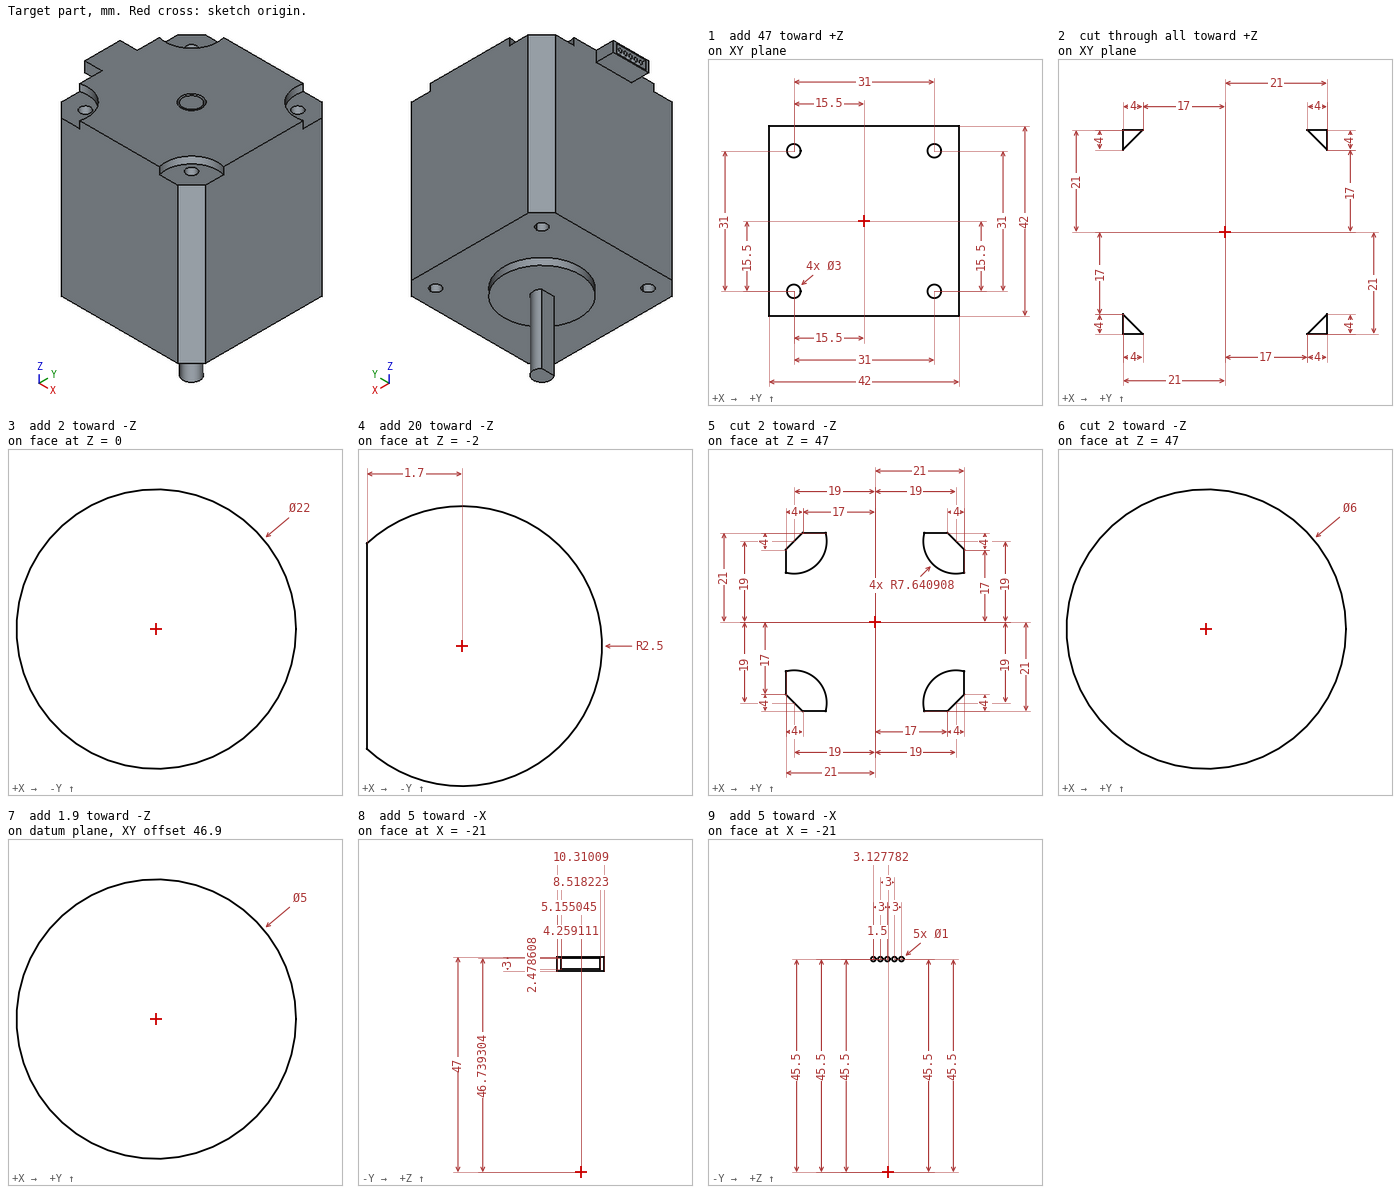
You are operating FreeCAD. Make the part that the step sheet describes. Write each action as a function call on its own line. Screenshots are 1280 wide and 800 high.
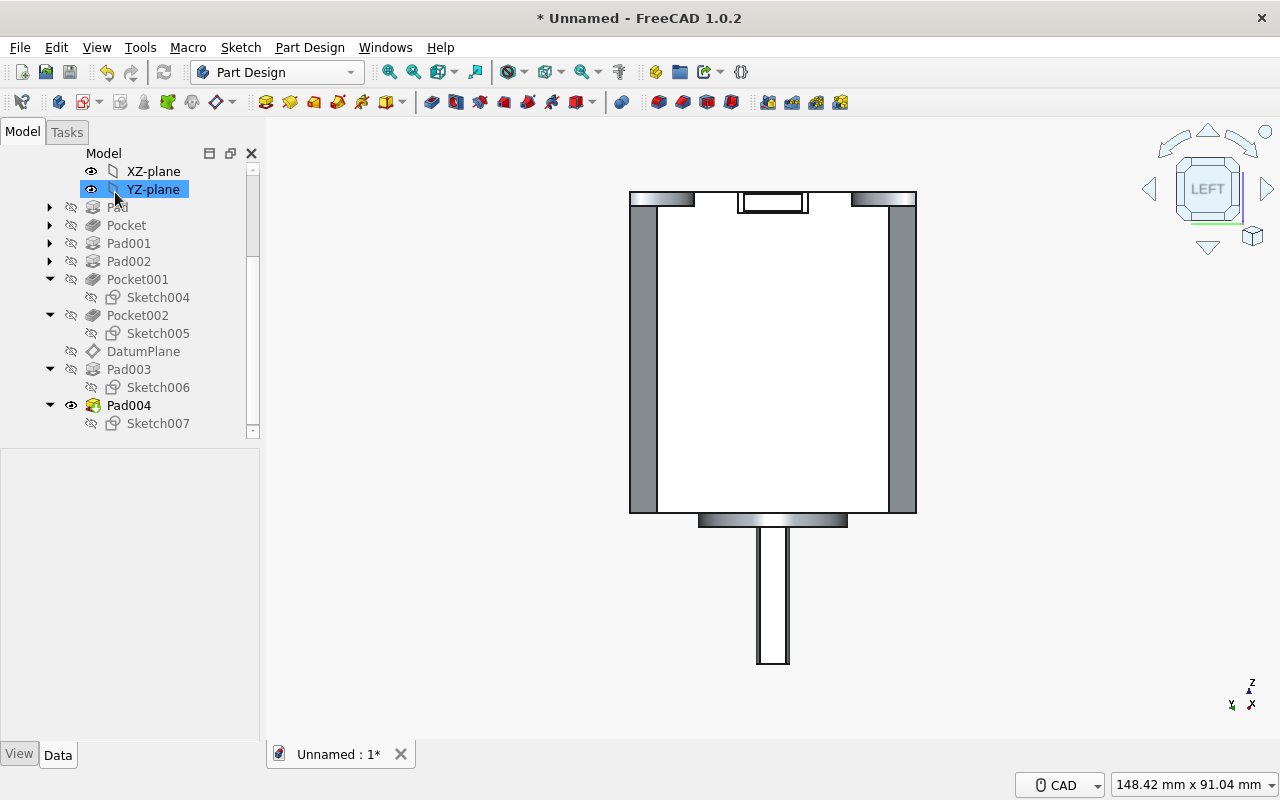
click(773, 352)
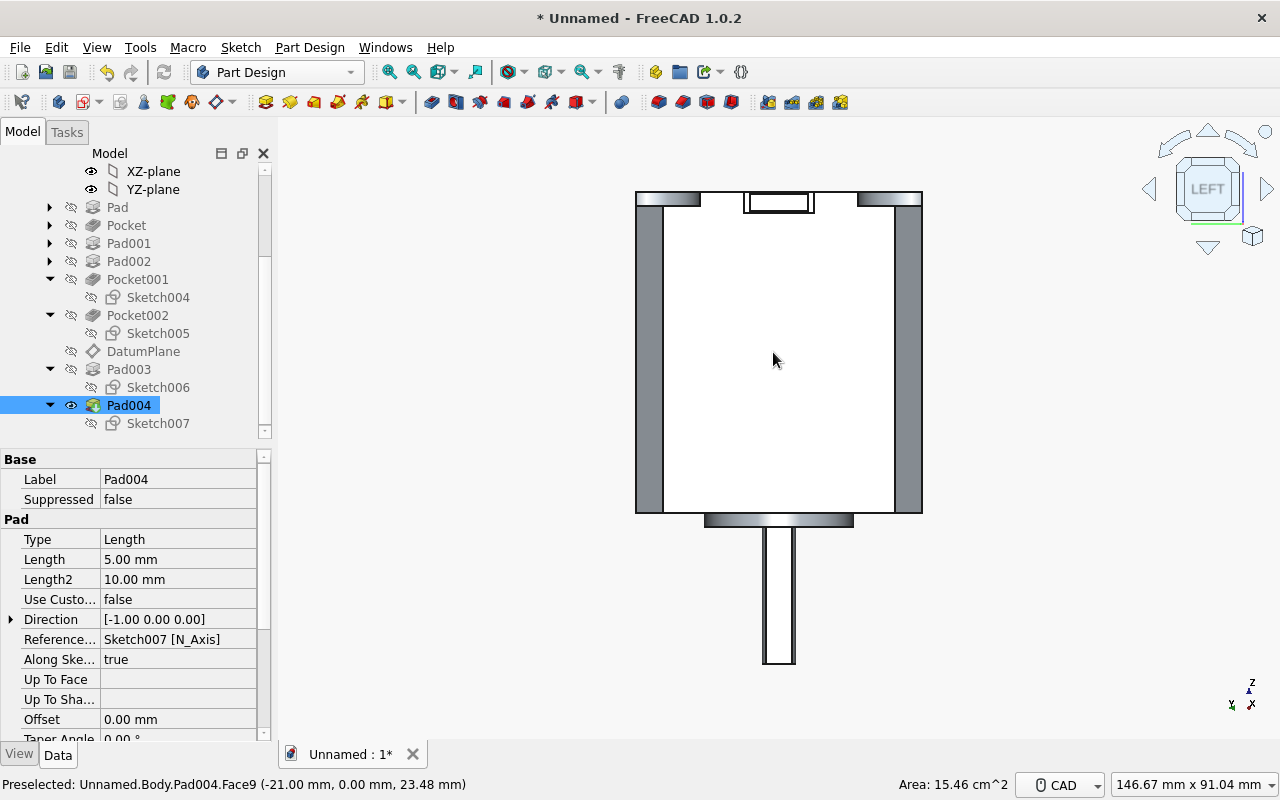
click(84, 102)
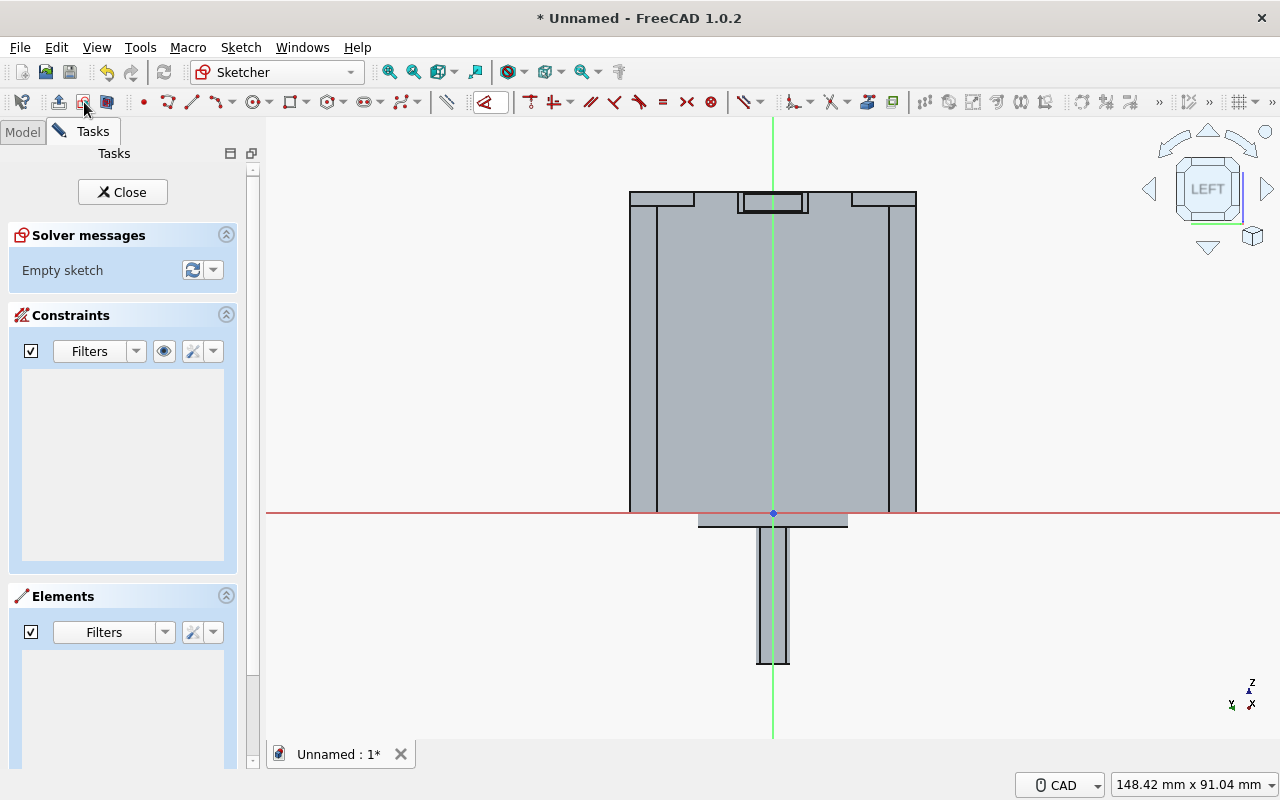
scroll(779, 180, up, 12)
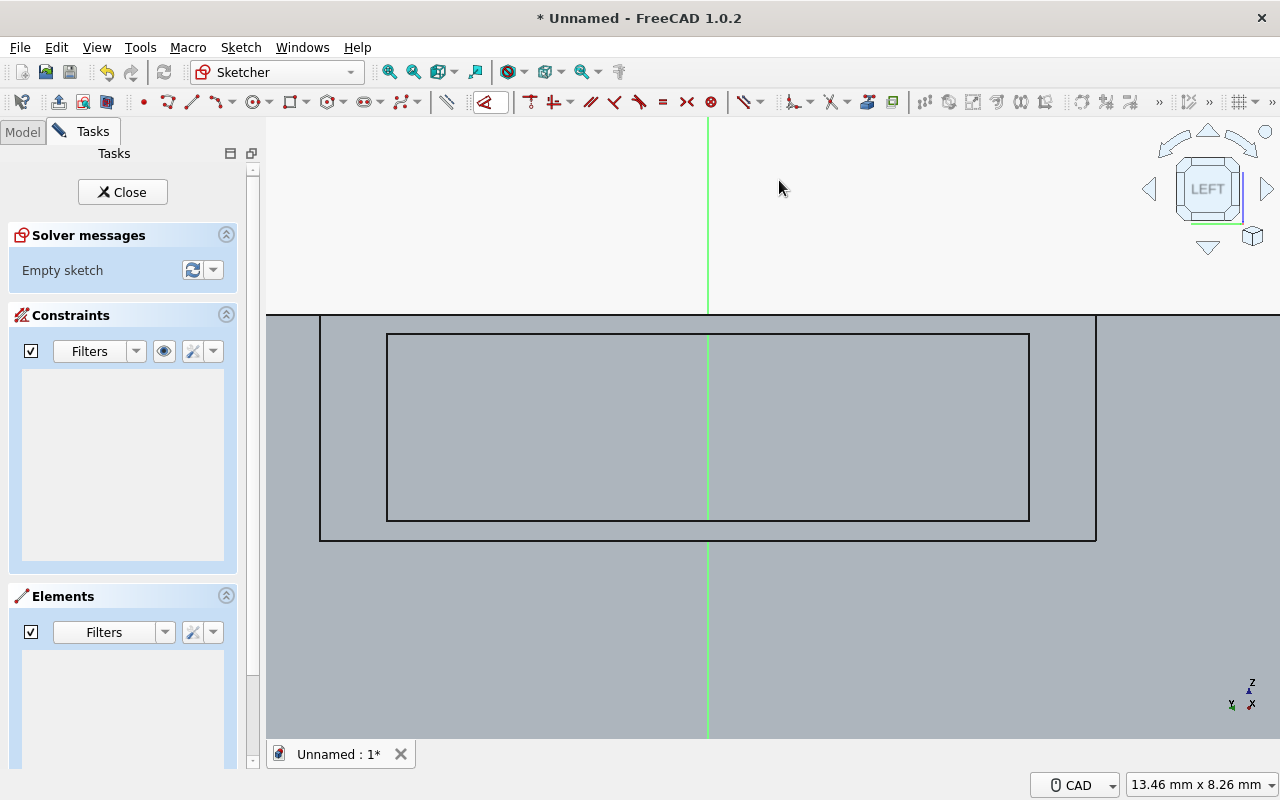
click(254, 102)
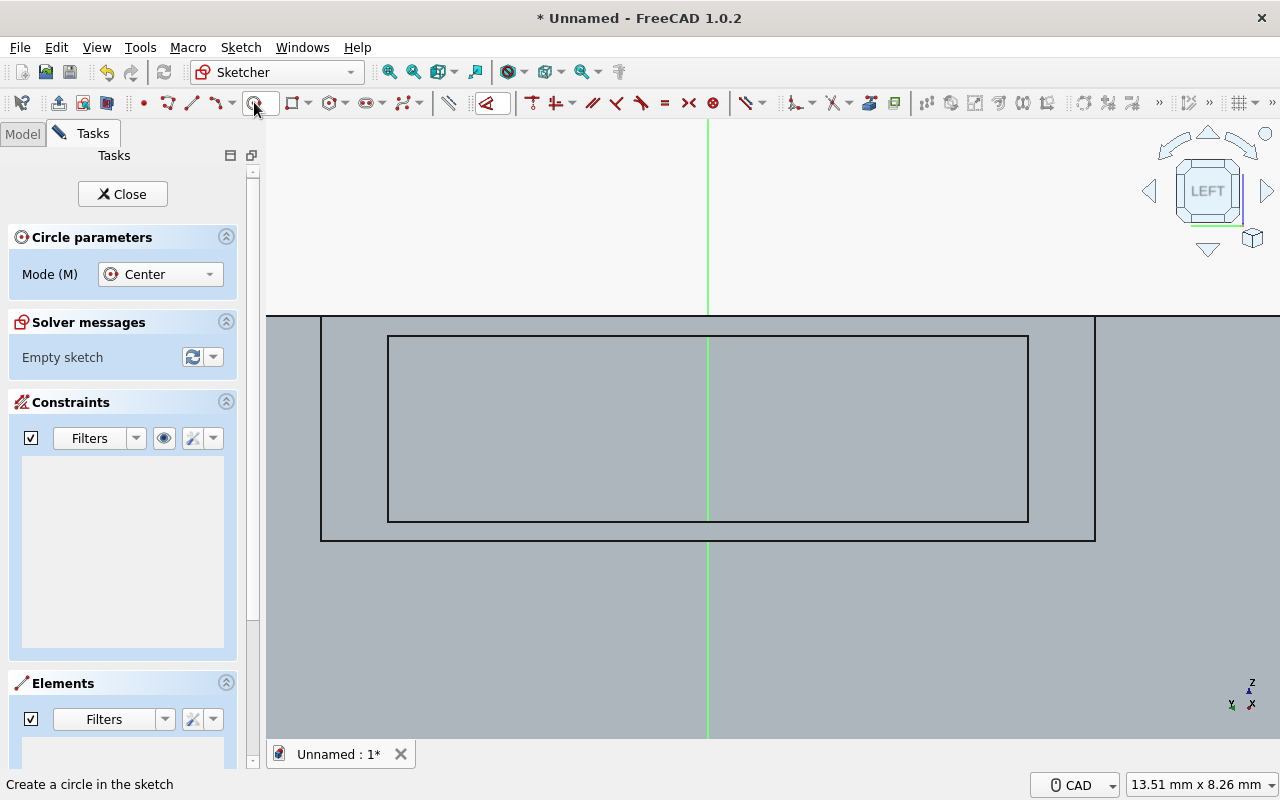
click(473, 429)
click(500, 402)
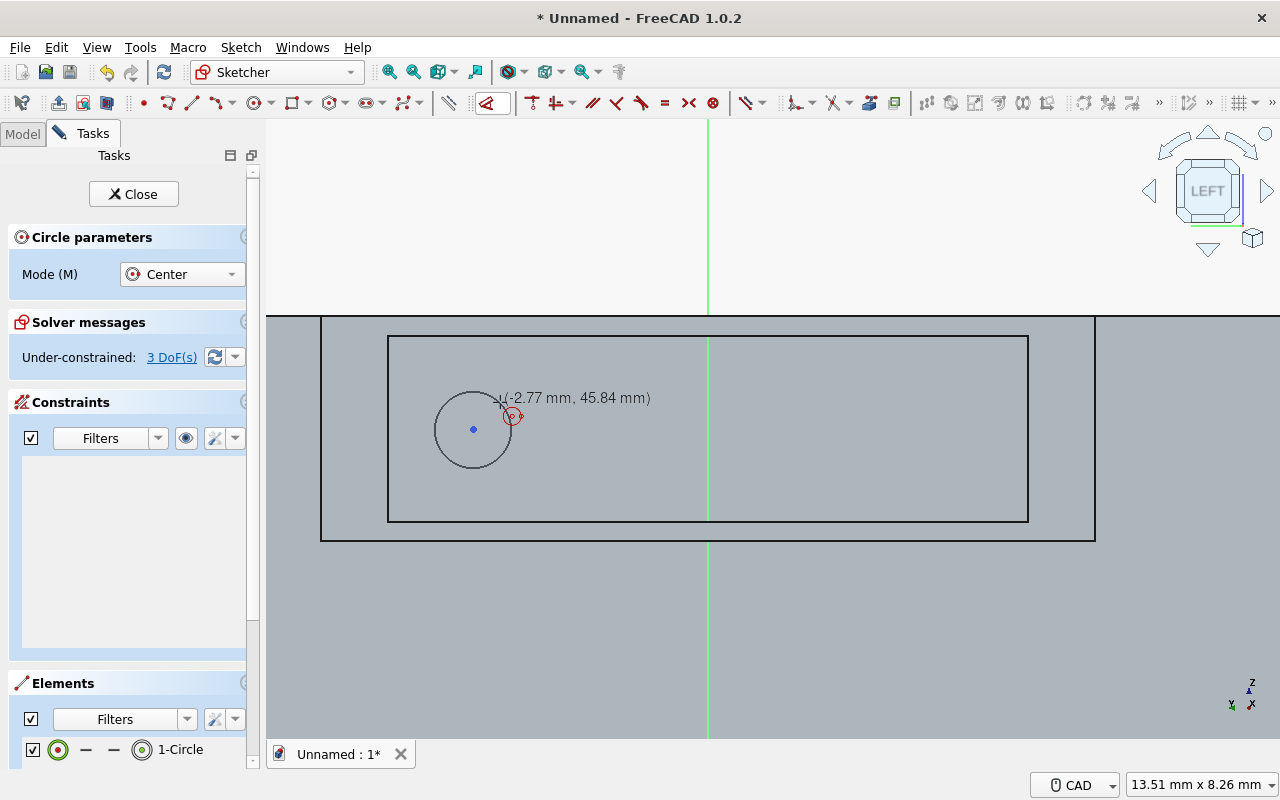
click(586, 429)
click(612, 402)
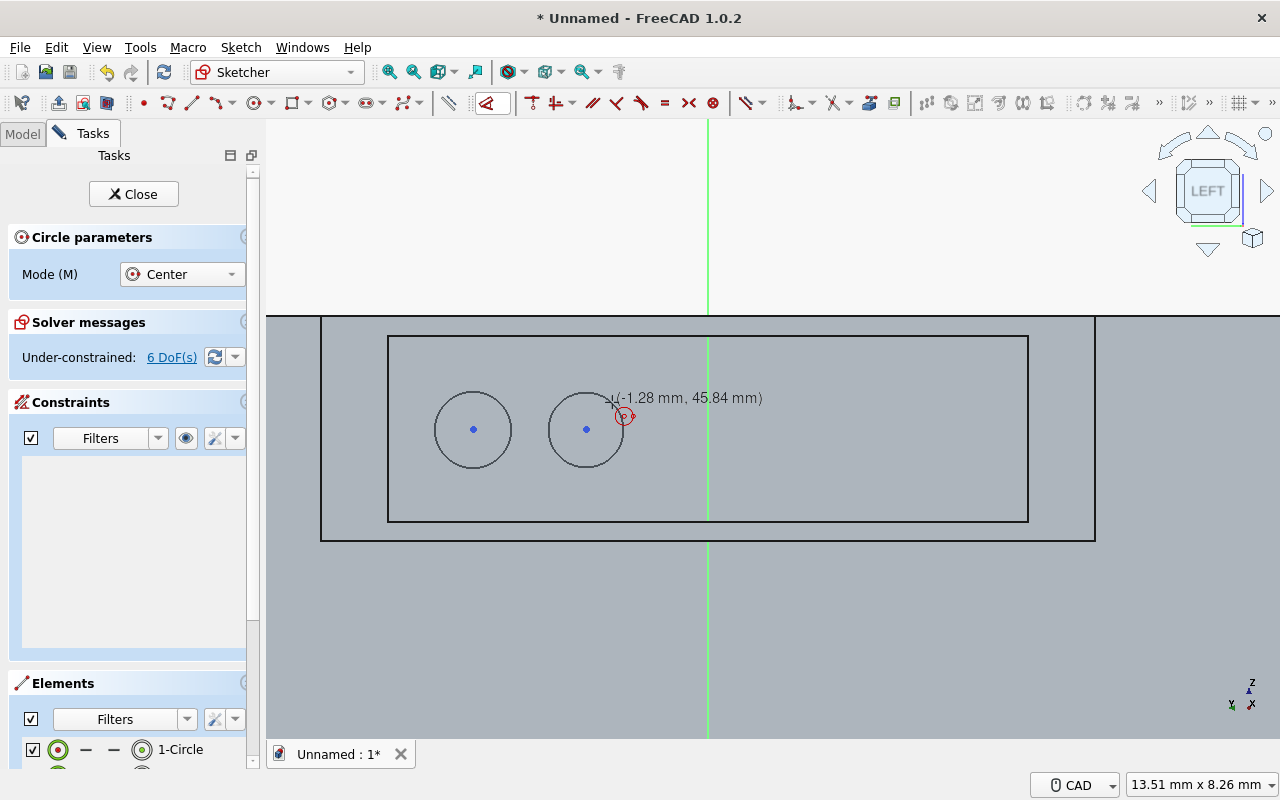
scroll(698, 429, up, 3)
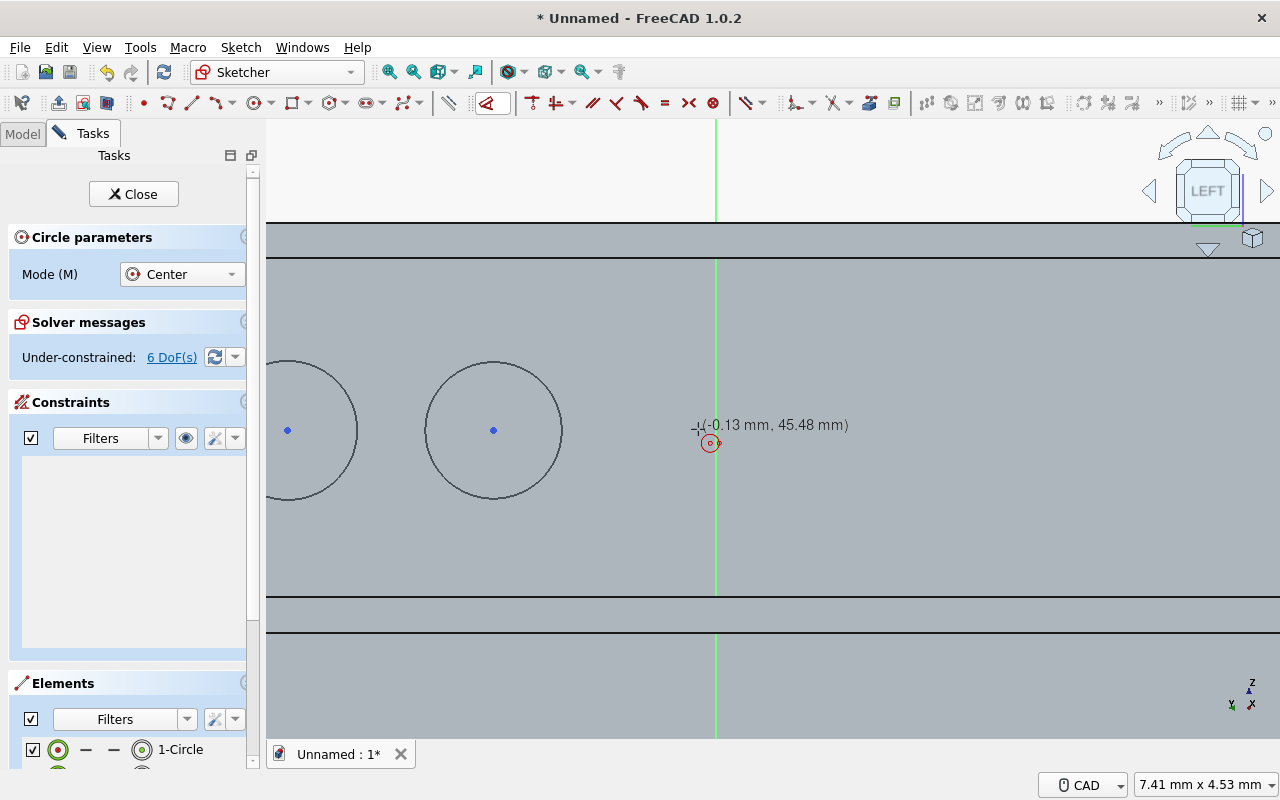
click(698, 428)
click(747, 379)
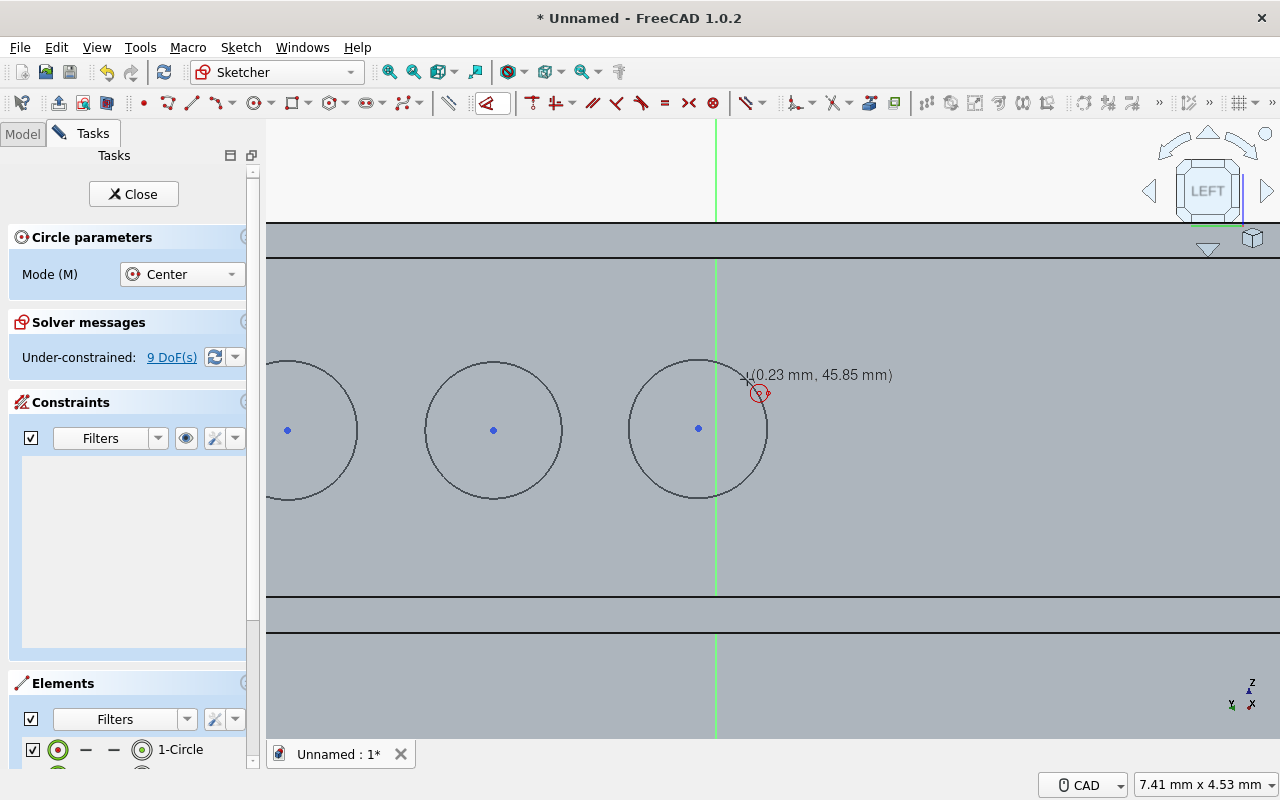
click(904, 428)
click(952, 379)